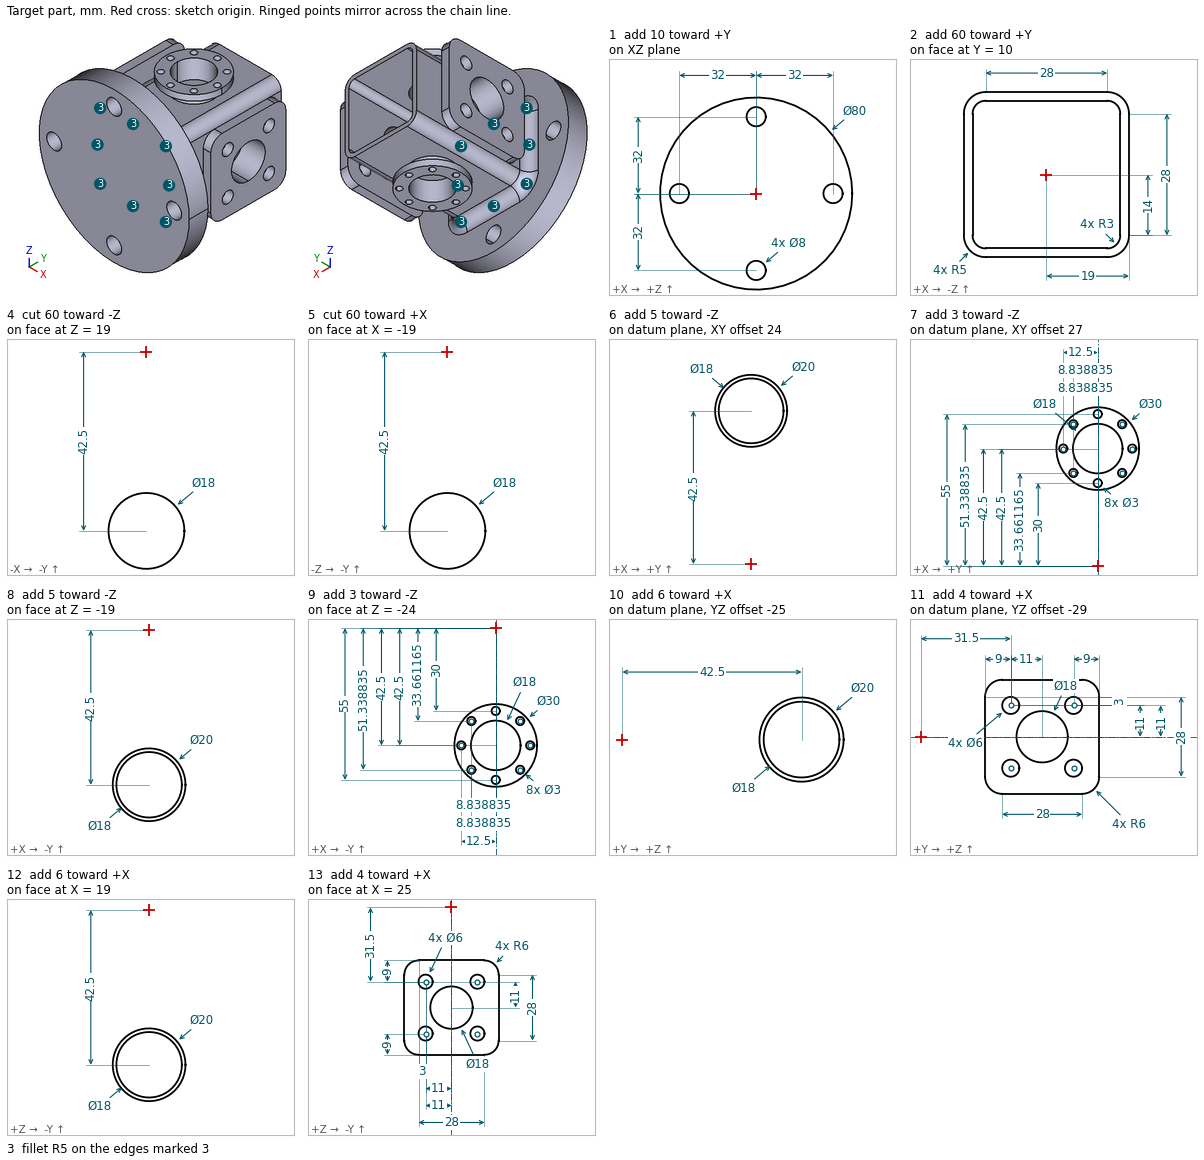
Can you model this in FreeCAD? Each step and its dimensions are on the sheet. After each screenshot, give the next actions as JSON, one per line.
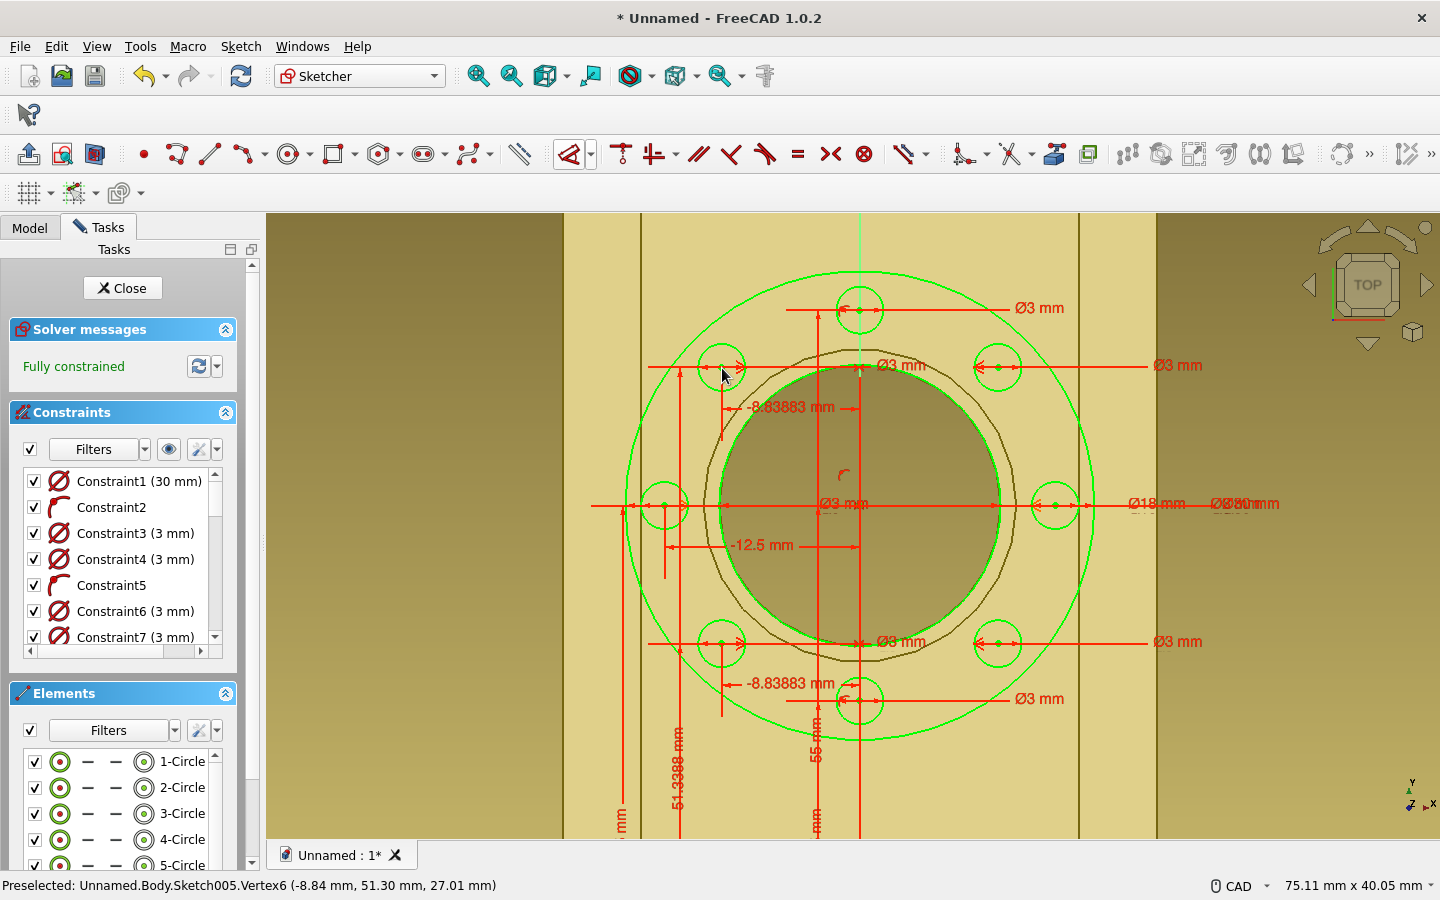
{"action": "left_click", "coordinate": [123, 288]}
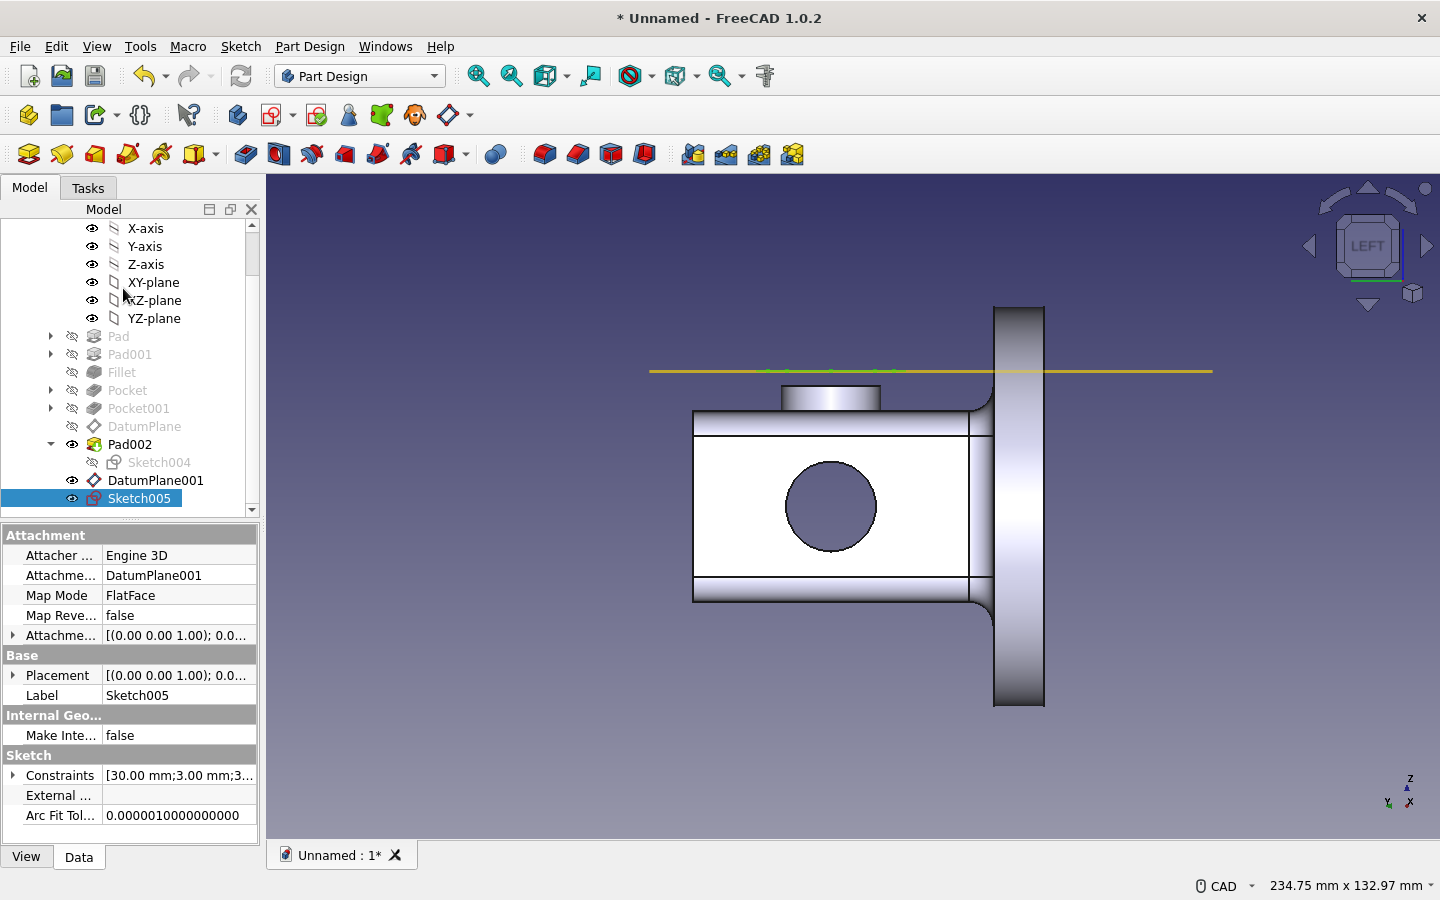
{"action": "left_click", "coordinate": [29, 154]}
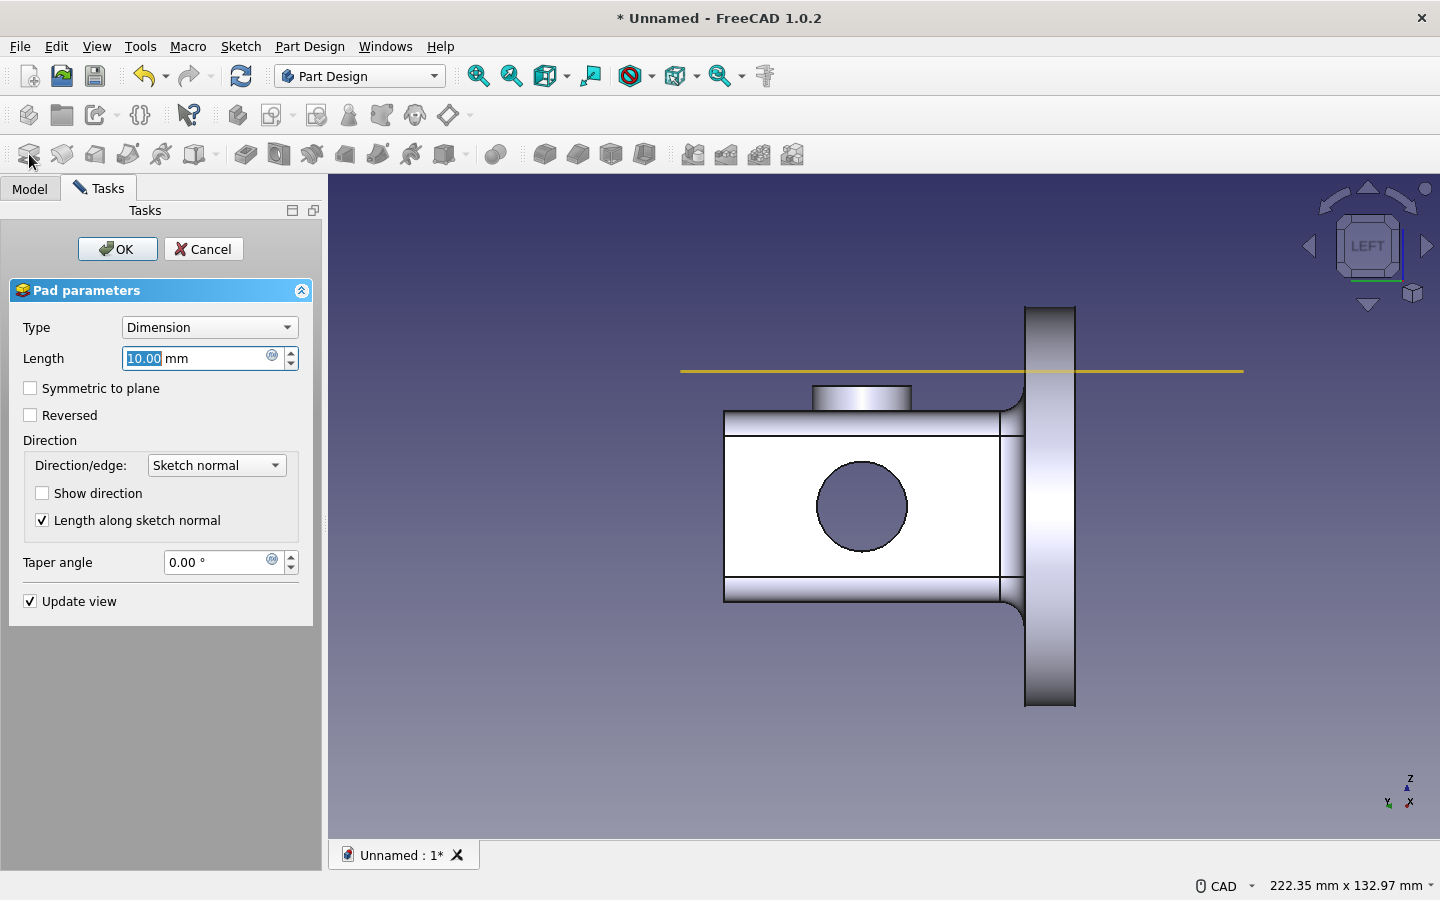
{"action": "type", "text": "3"}
{"action": "key", "text": "Tab"}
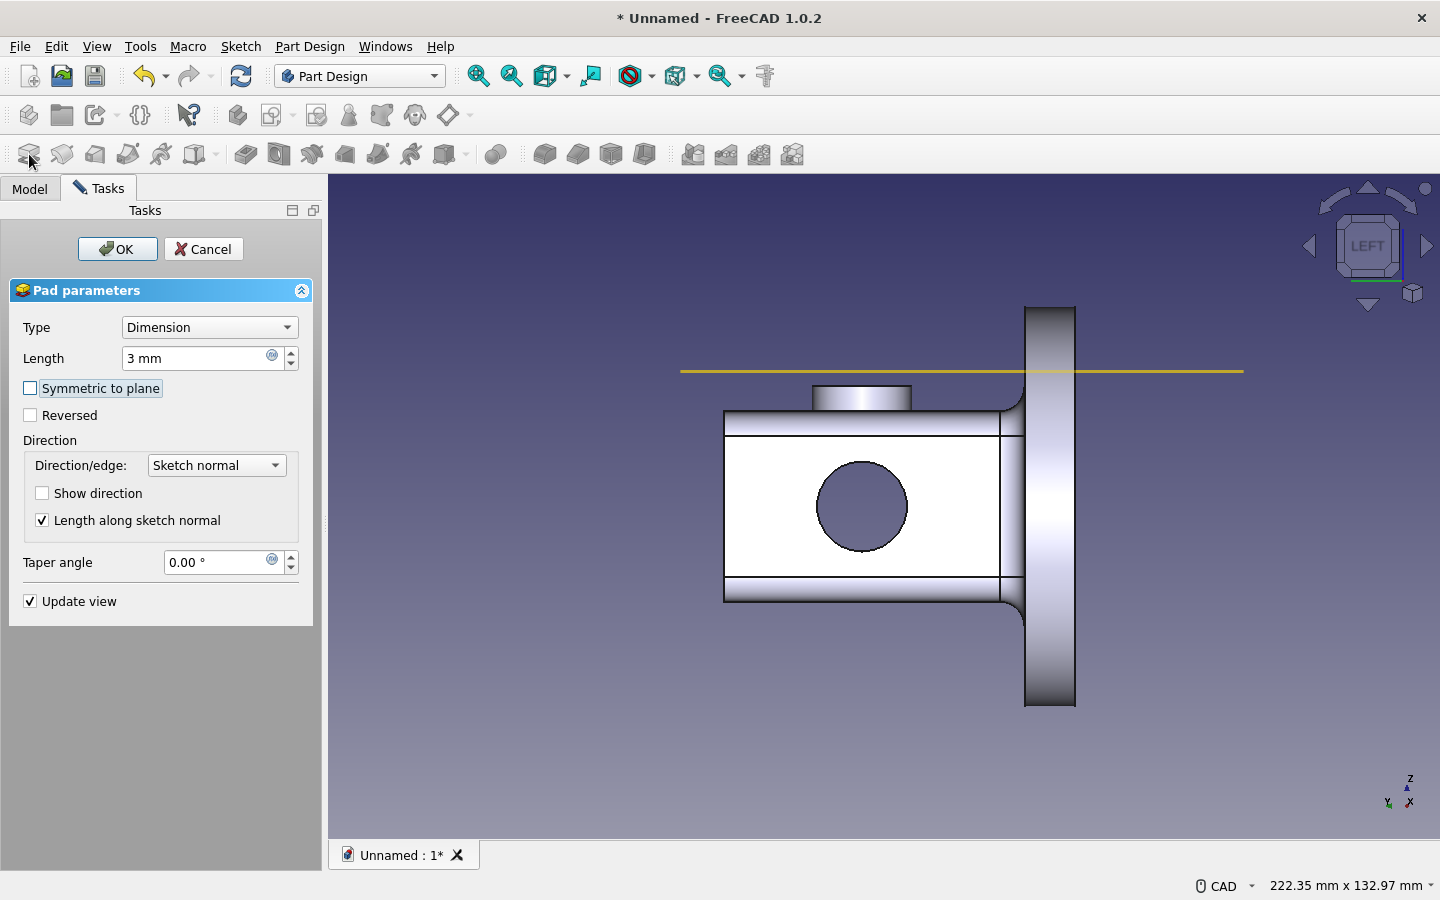
{"action": "left_click", "coordinate": [31, 415]}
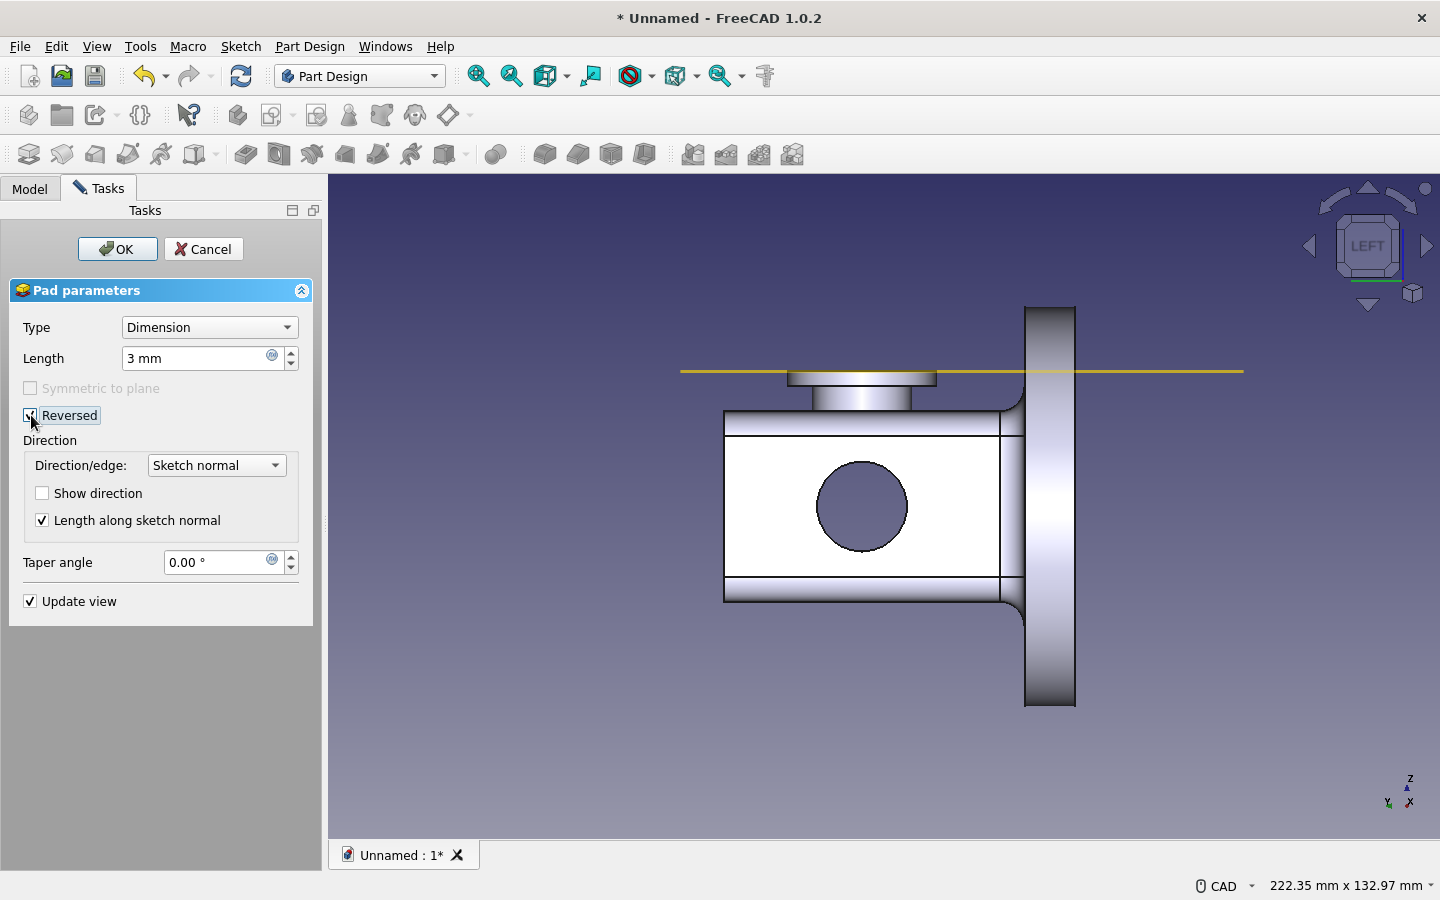
{"action": "left_click", "coordinate": [118, 249]}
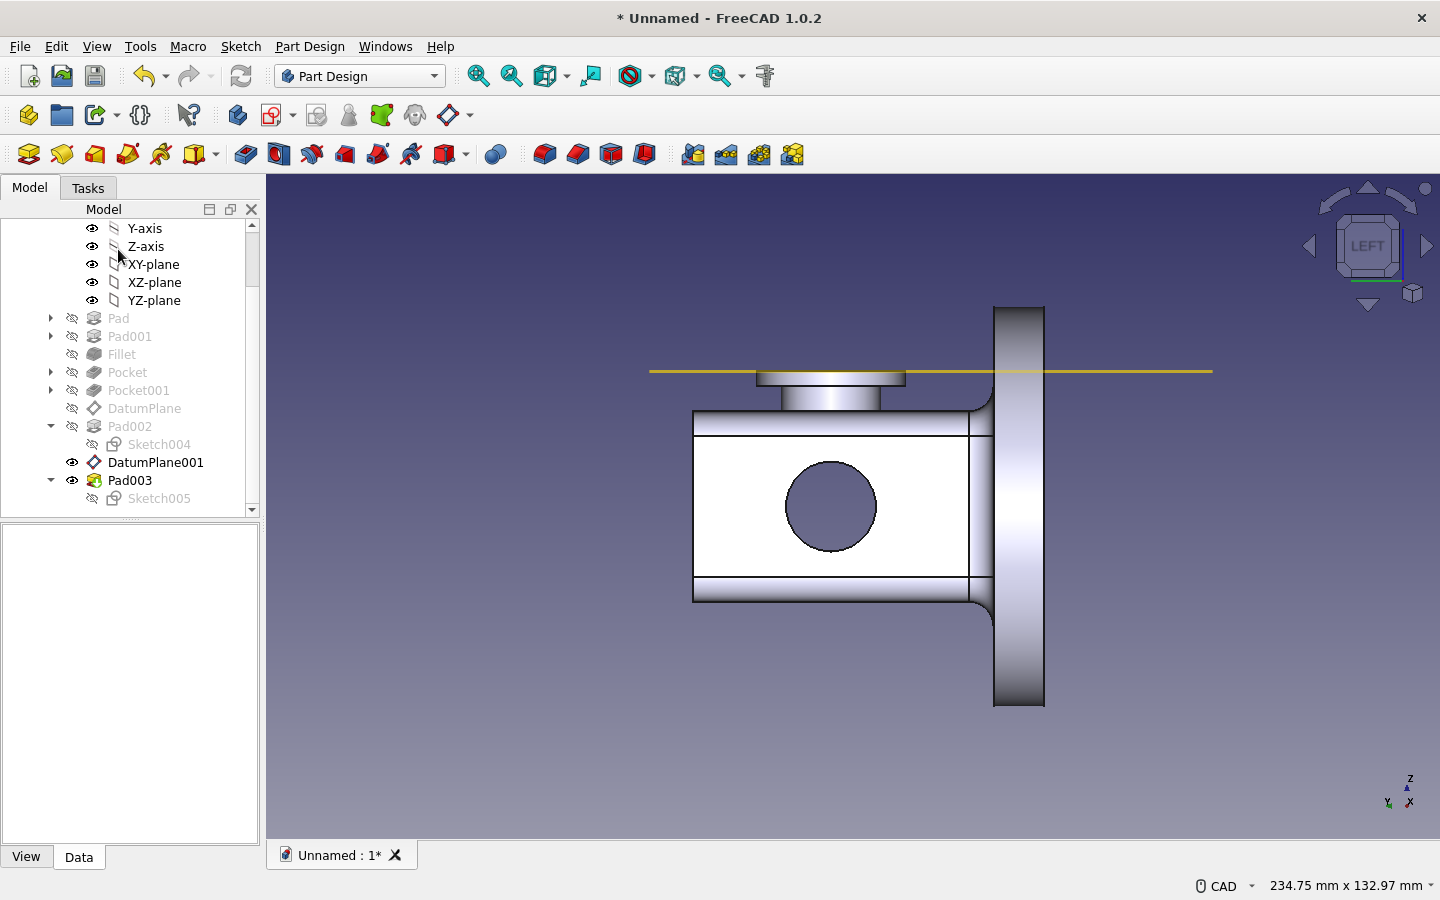
{"action": "left_click", "coordinate": [117, 462]}
{"action": "key", "text": "space"}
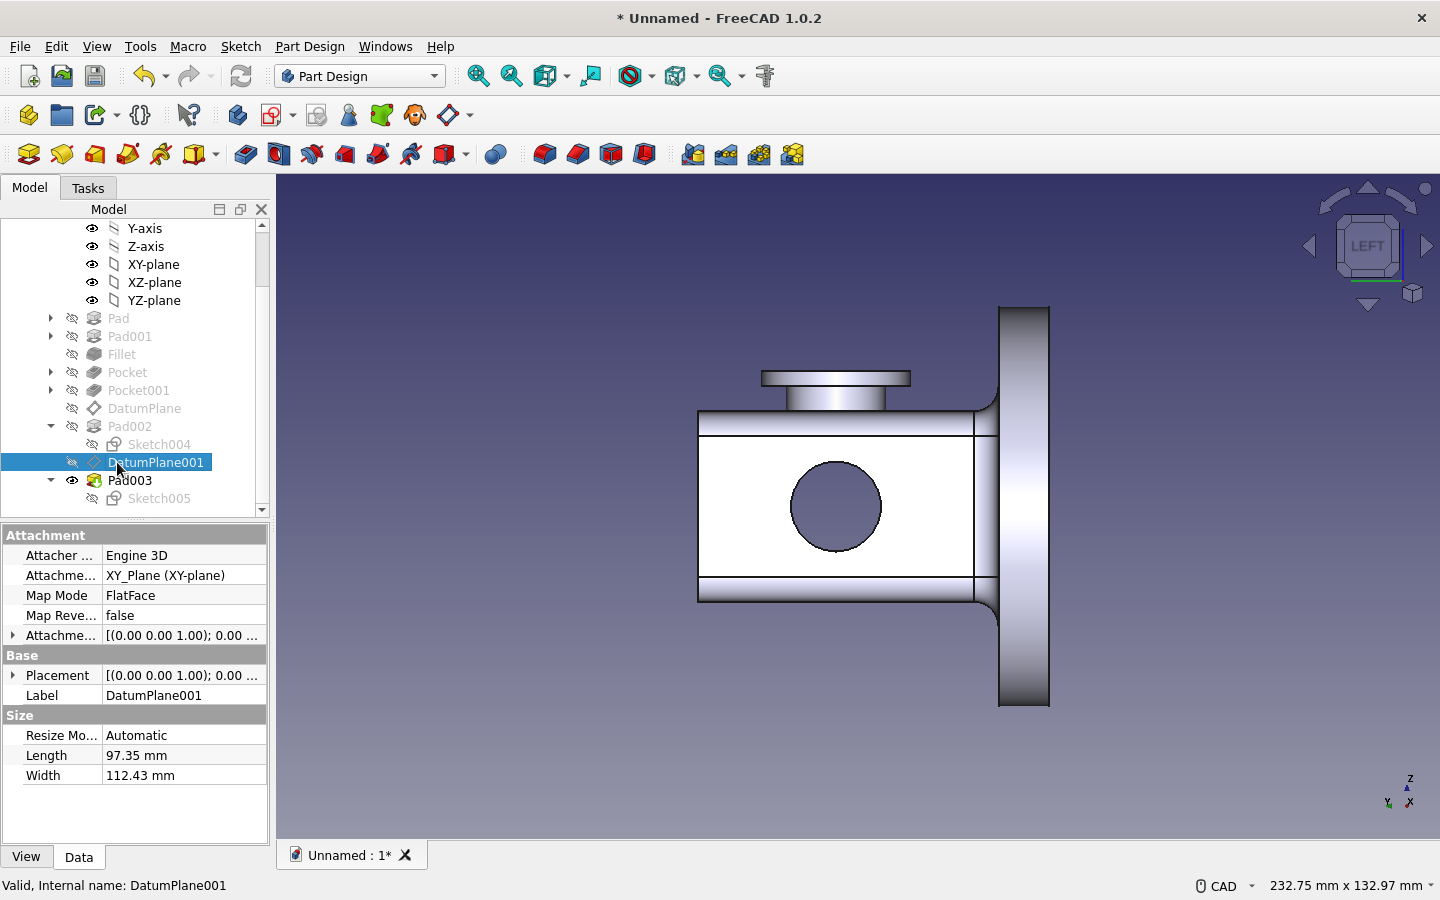
{"action": "key", "text": "5"}